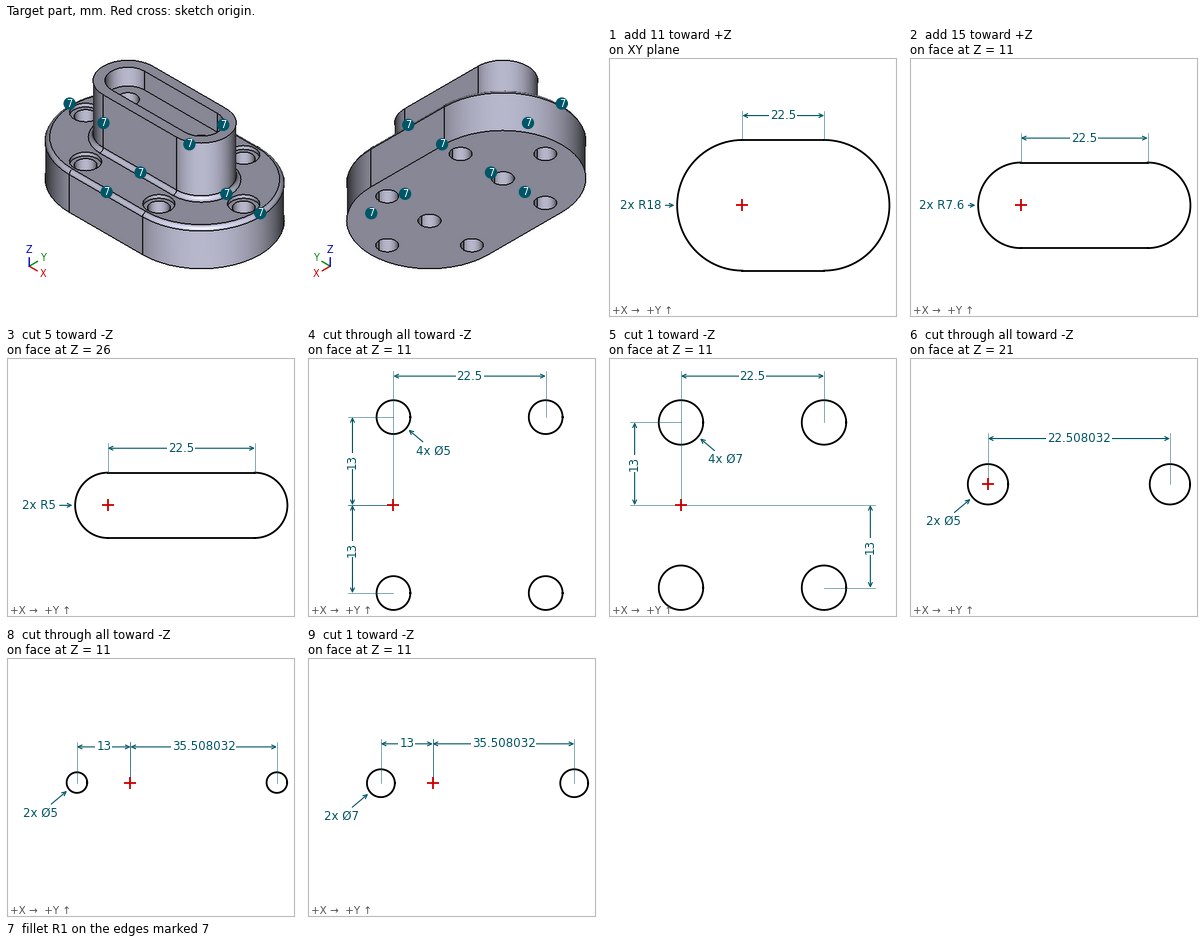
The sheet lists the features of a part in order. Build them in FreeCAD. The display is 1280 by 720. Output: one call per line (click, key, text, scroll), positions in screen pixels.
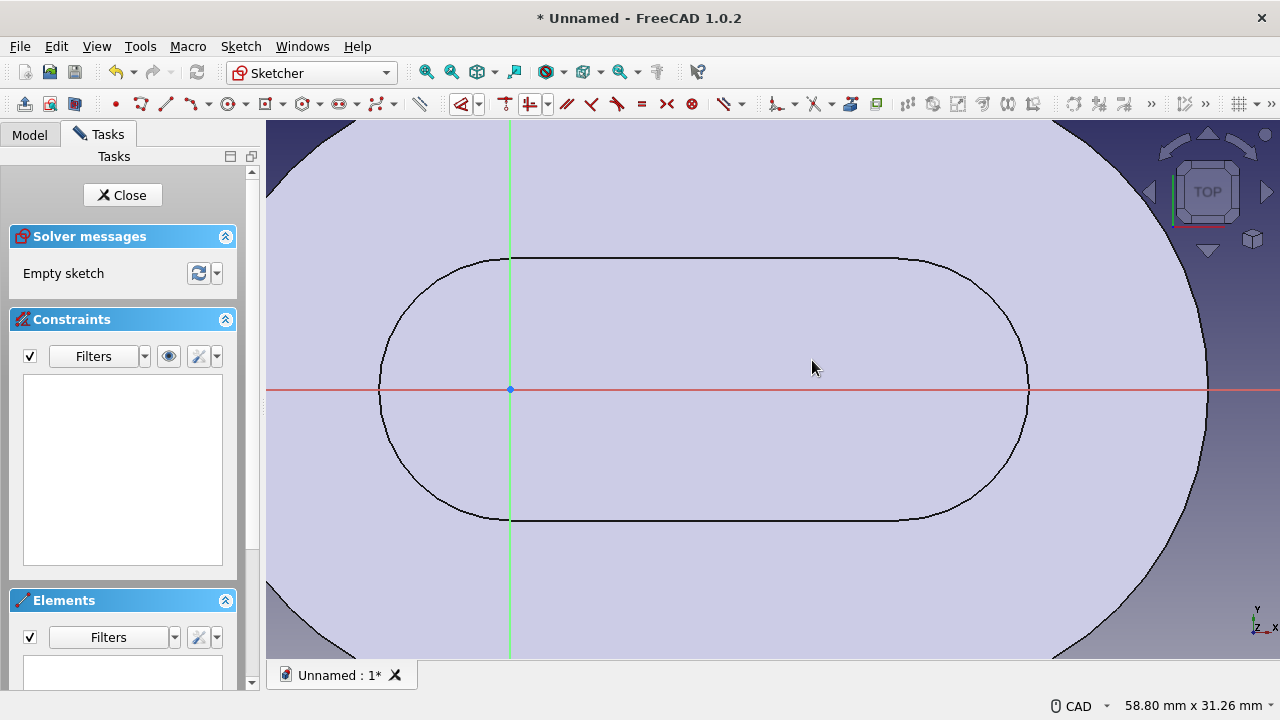
key(g)
key(s)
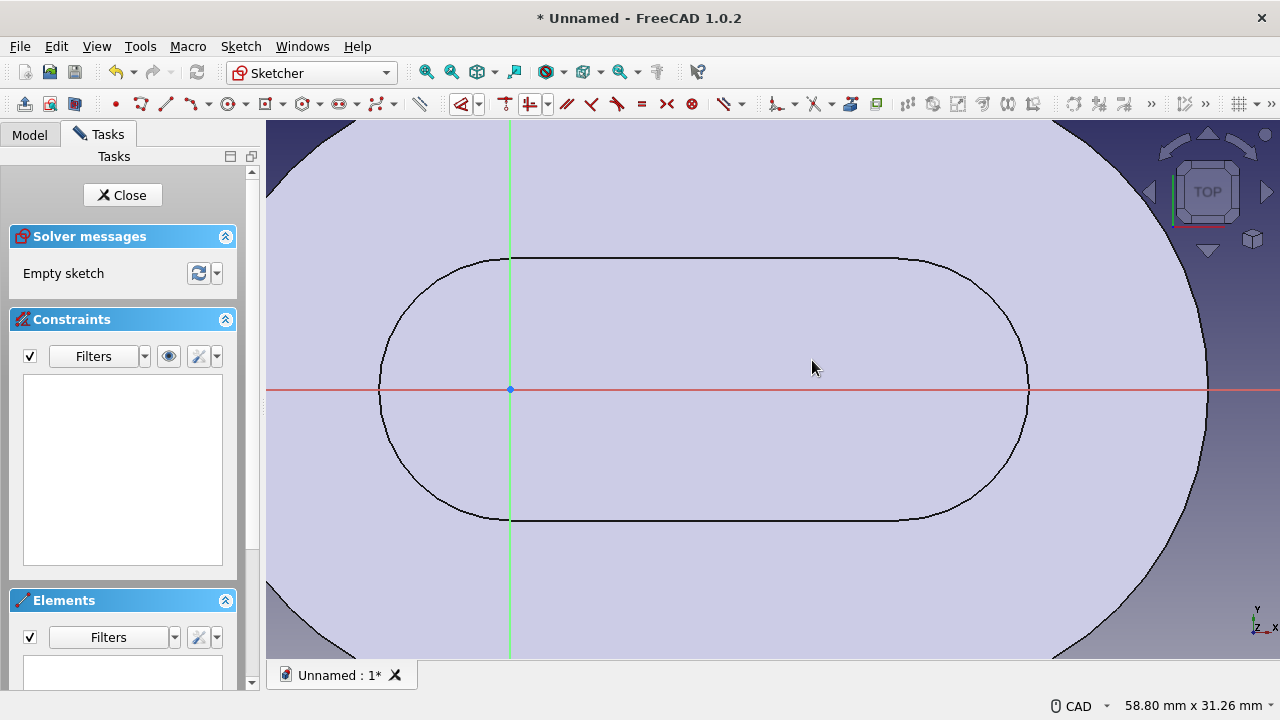
click(510, 390)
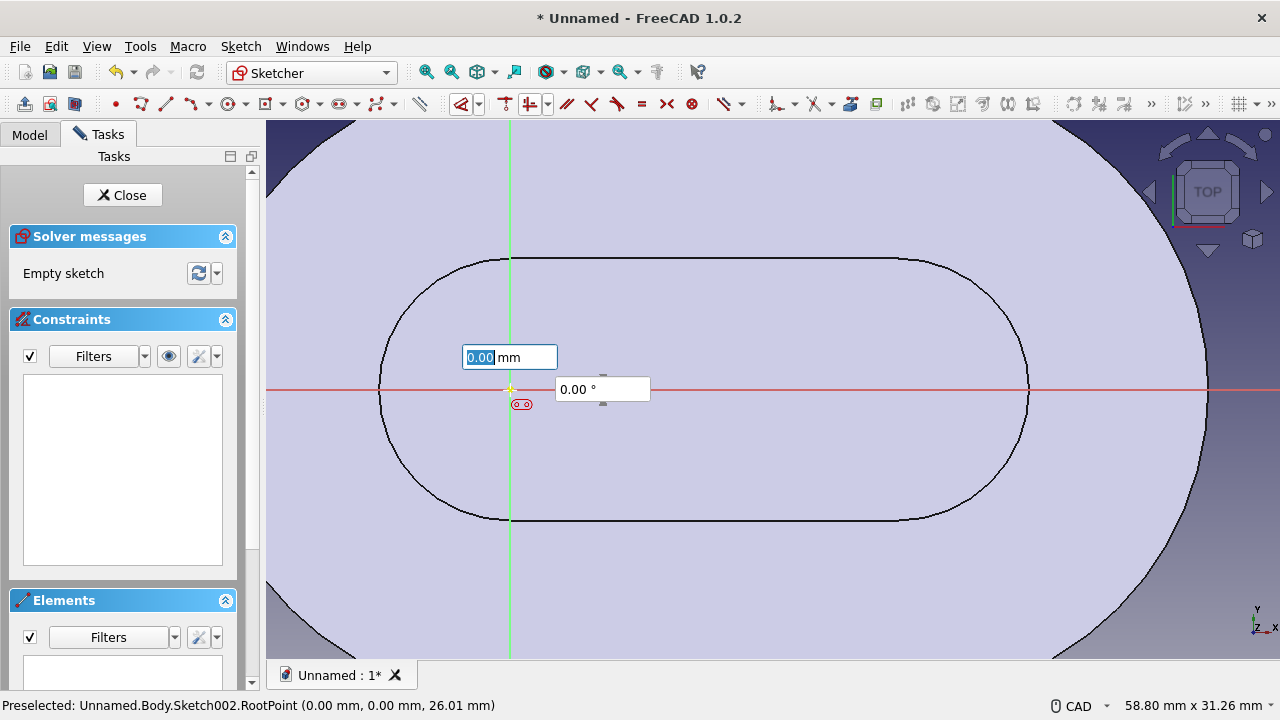
click(898, 381)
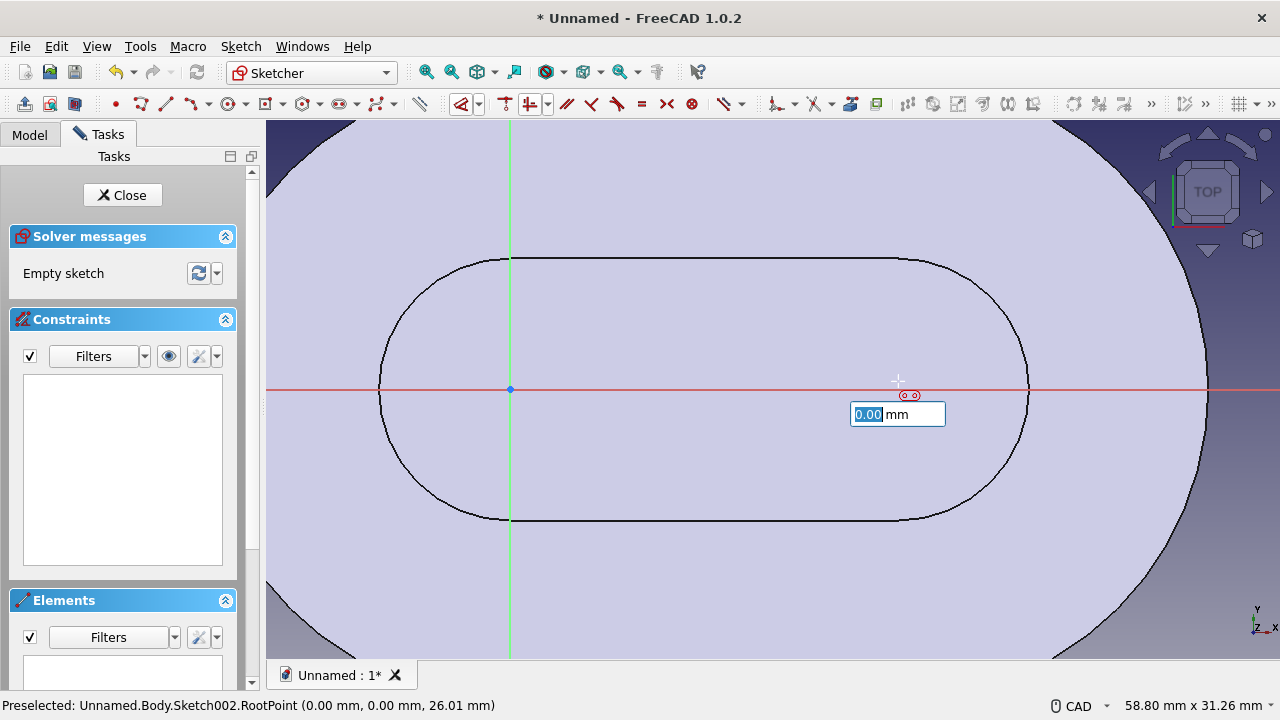
click(704, 303)
key(Escape)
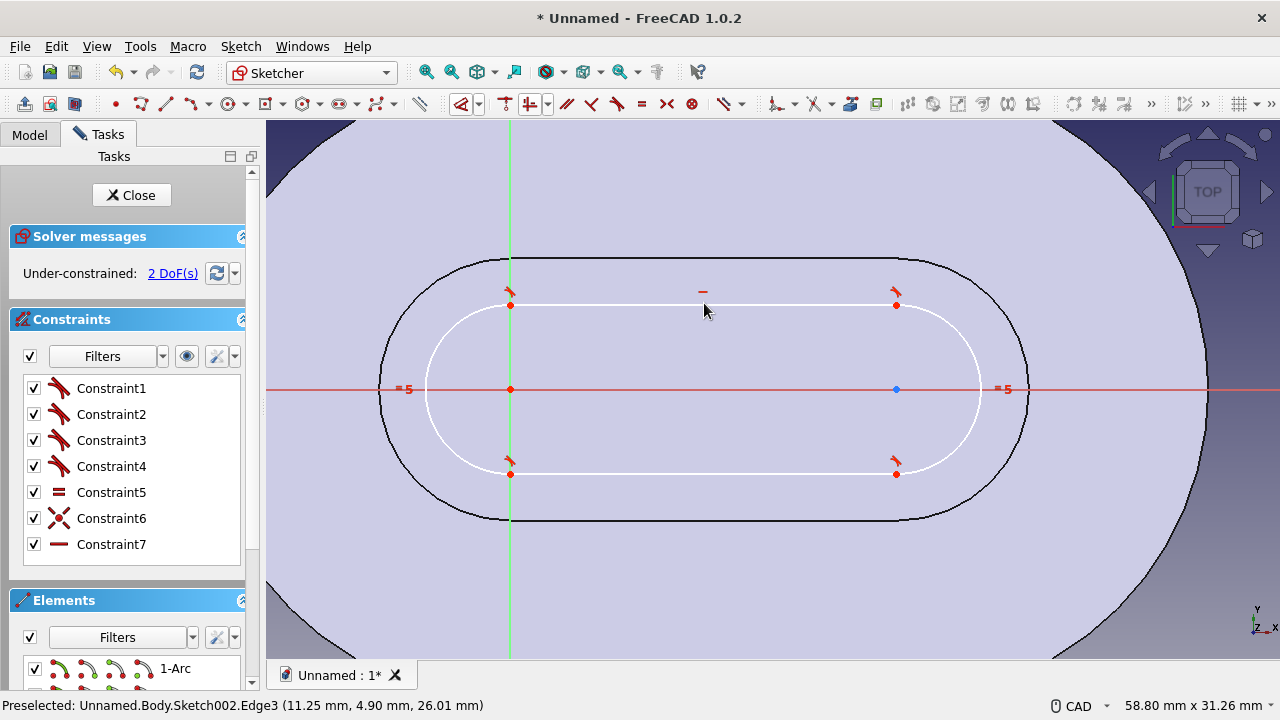
click(442, 340)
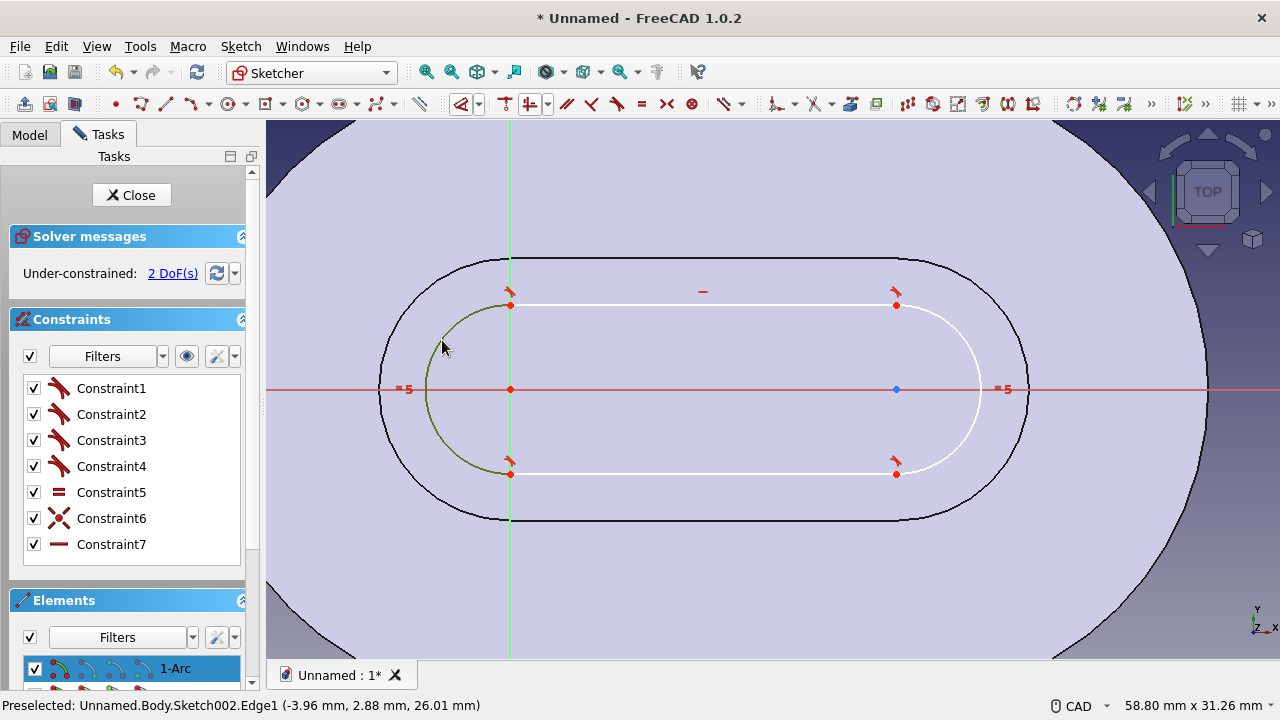
key(k)
key(r)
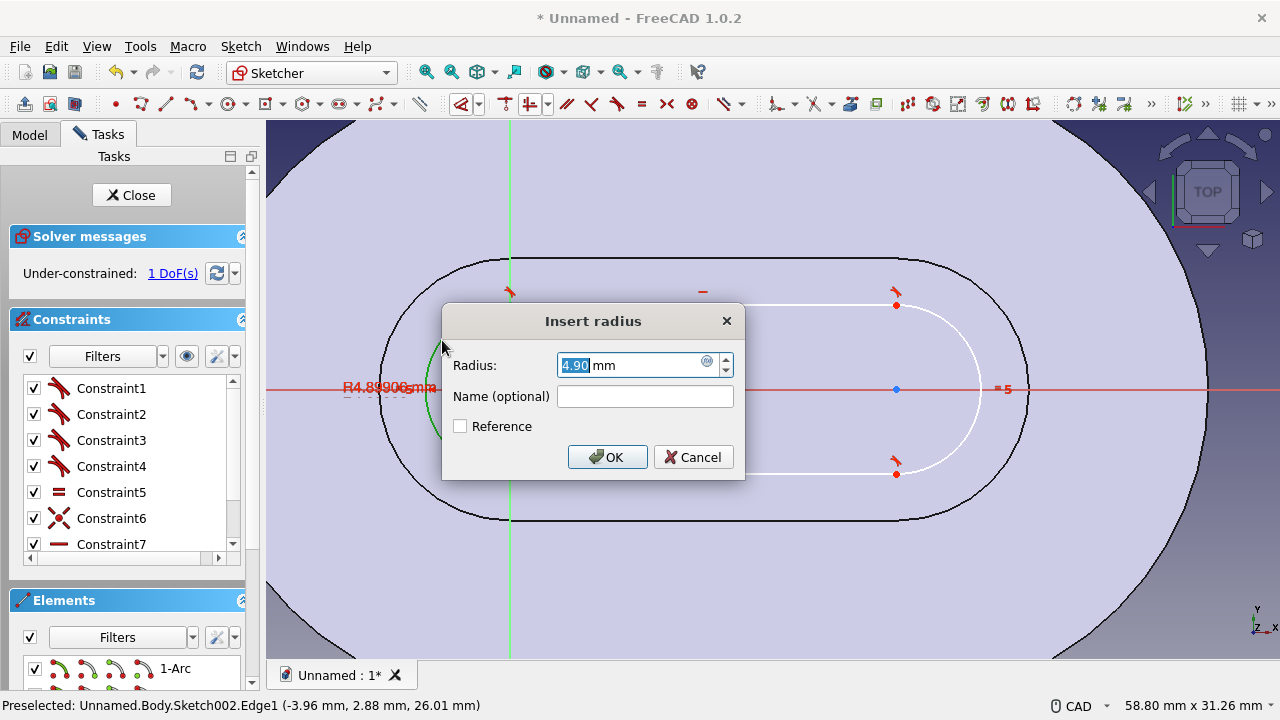
text(5)
key(Return)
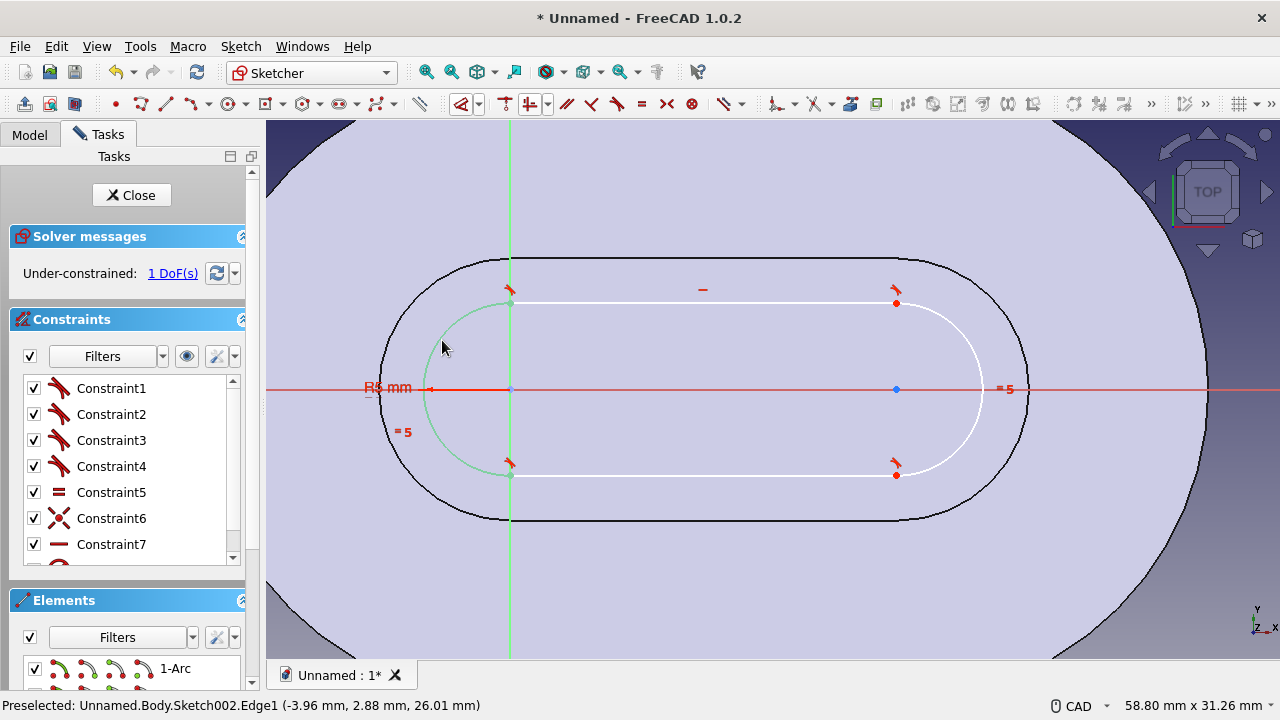
click(626, 303)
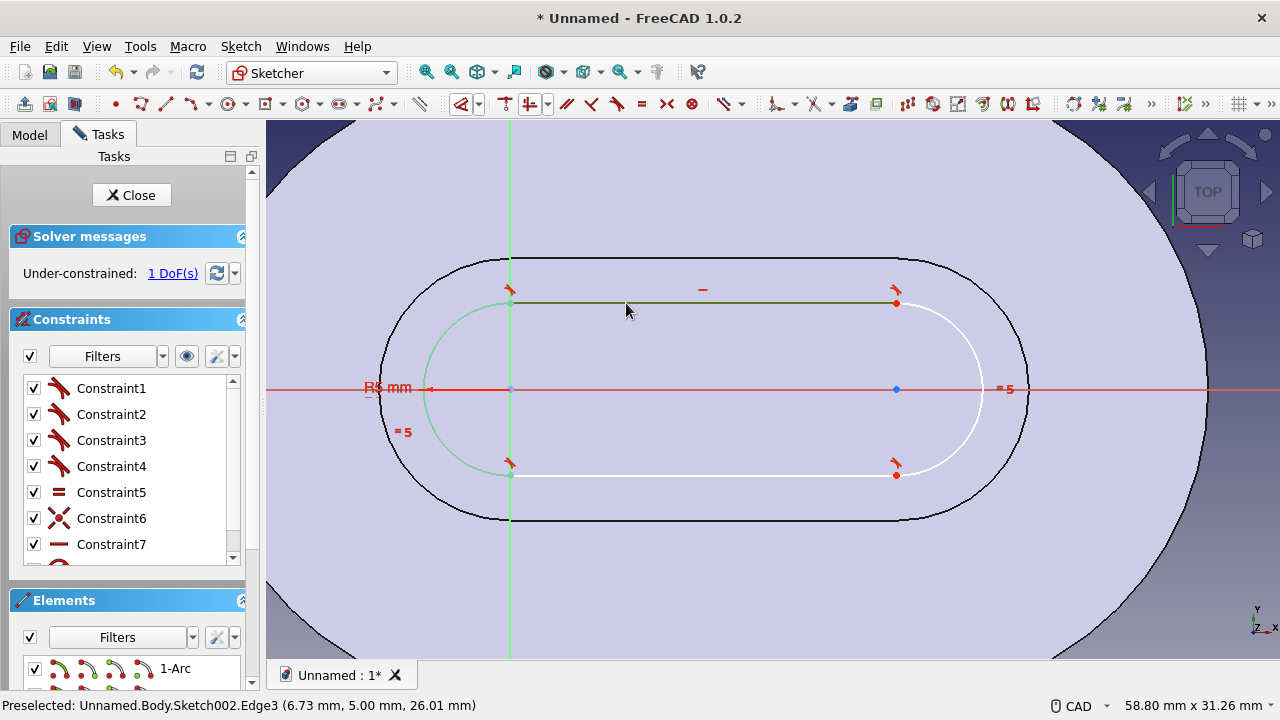
key(l)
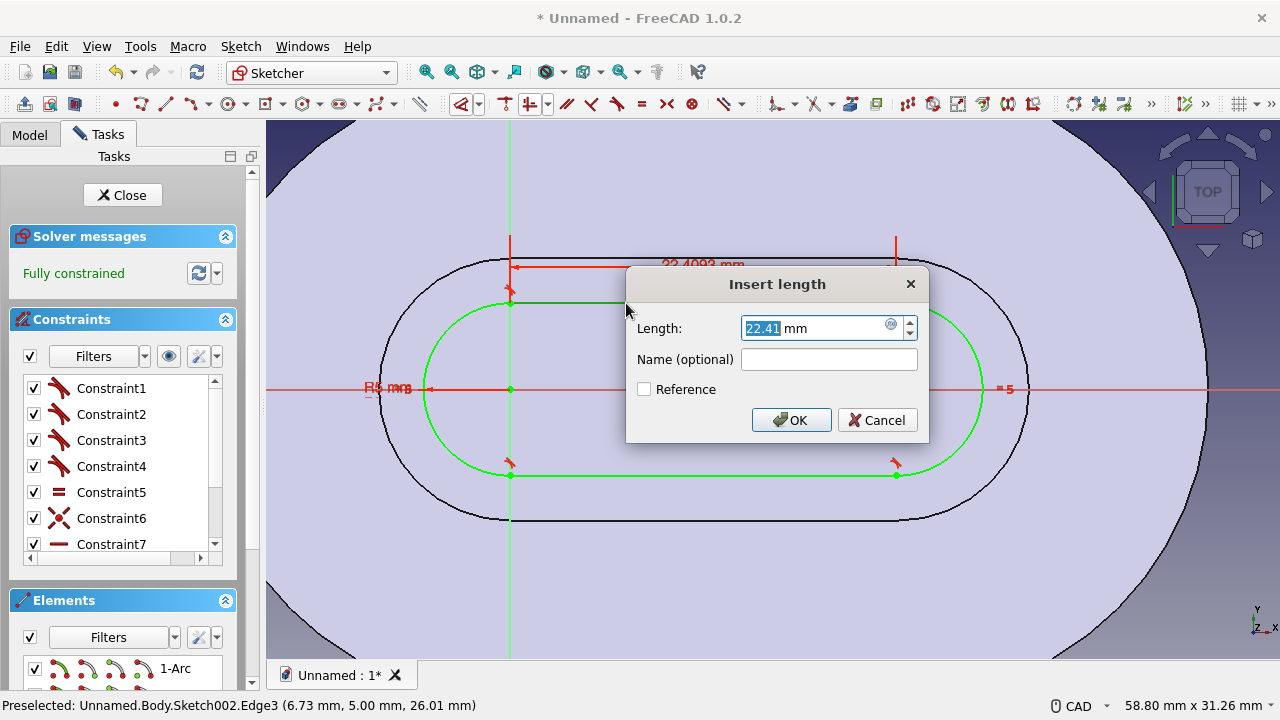
text(22.5)
key(Return)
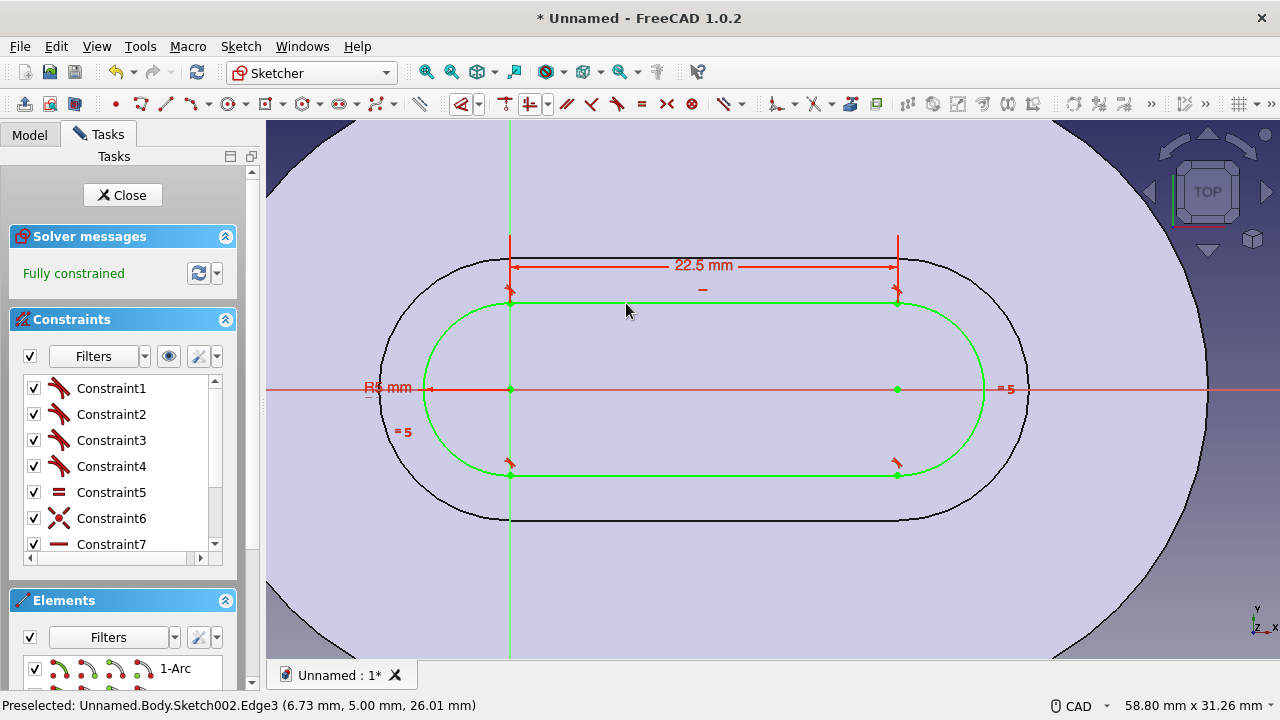
click(123, 195)